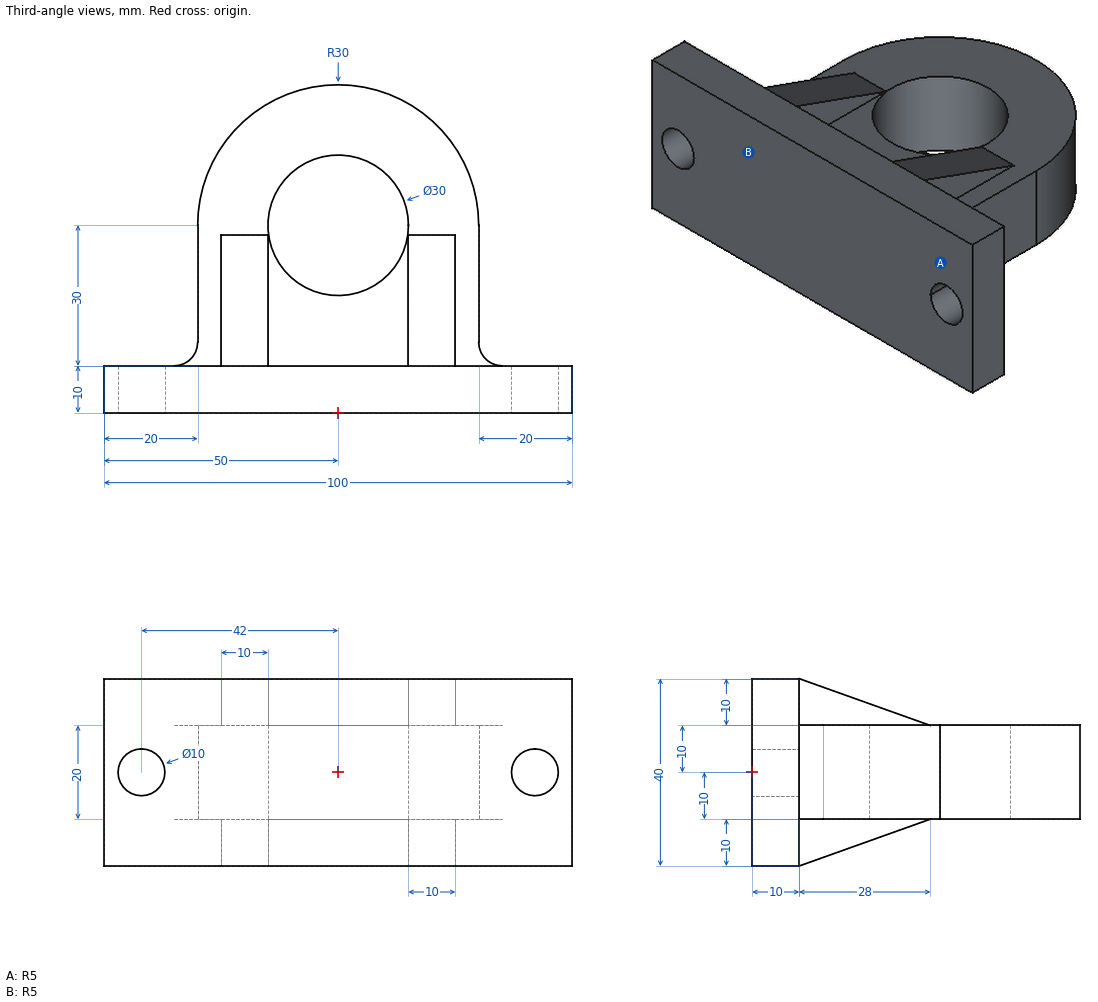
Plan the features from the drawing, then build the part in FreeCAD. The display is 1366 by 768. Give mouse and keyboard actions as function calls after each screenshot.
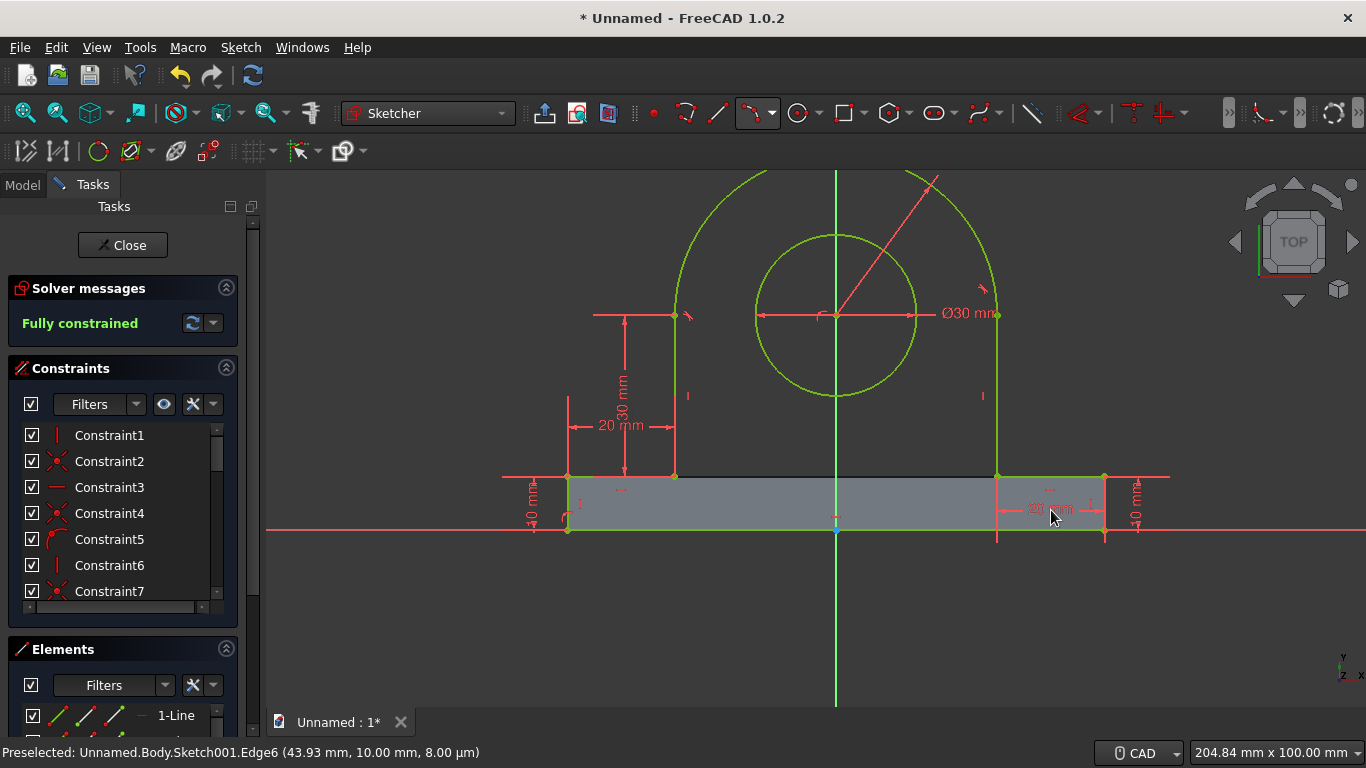
click(123, 245)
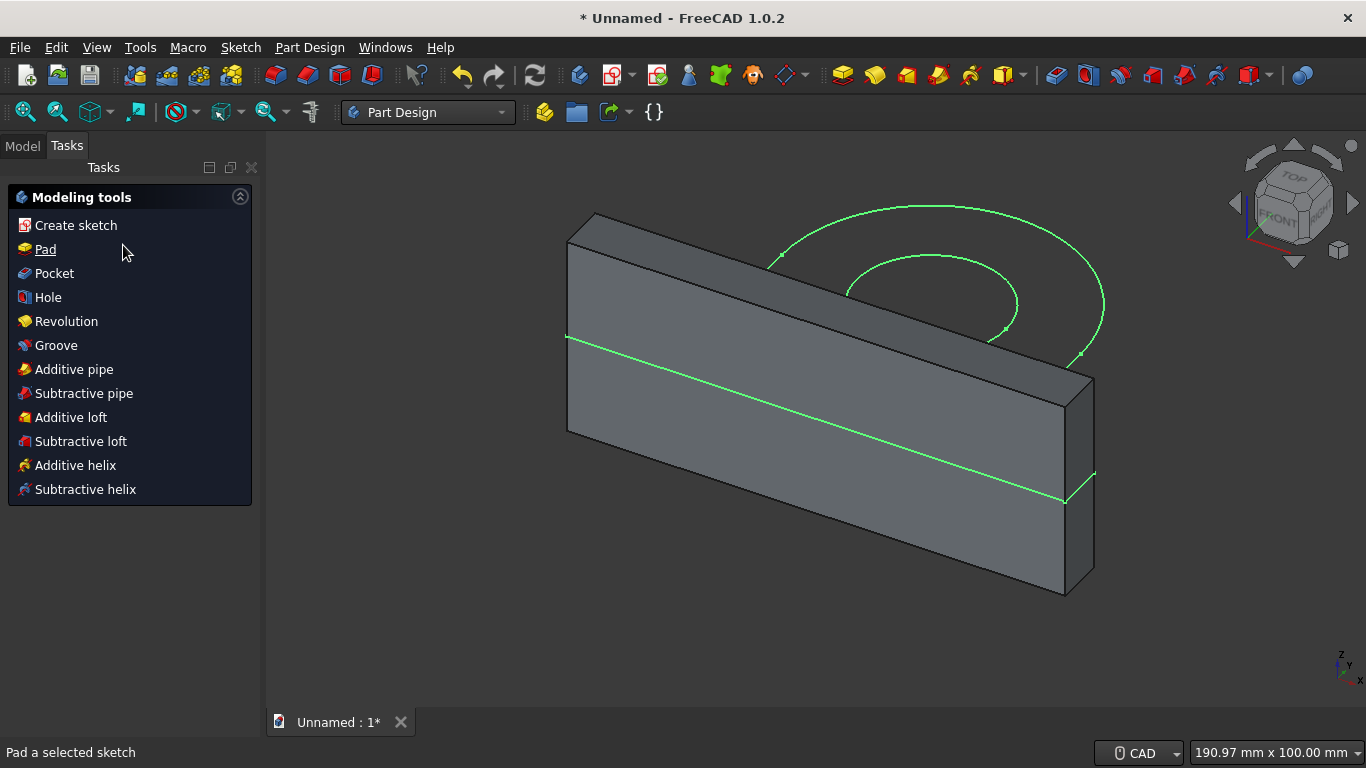
click(844, 76)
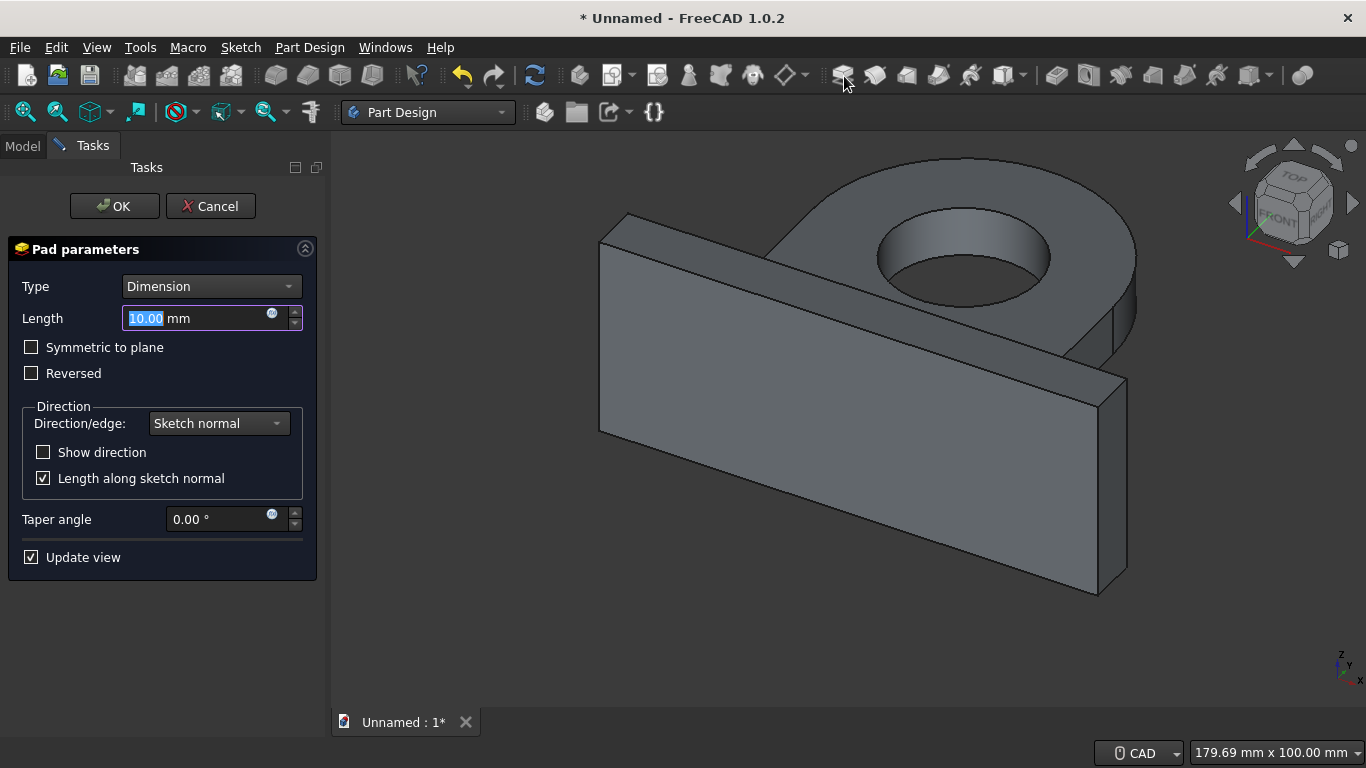
text(20)
key(Tab)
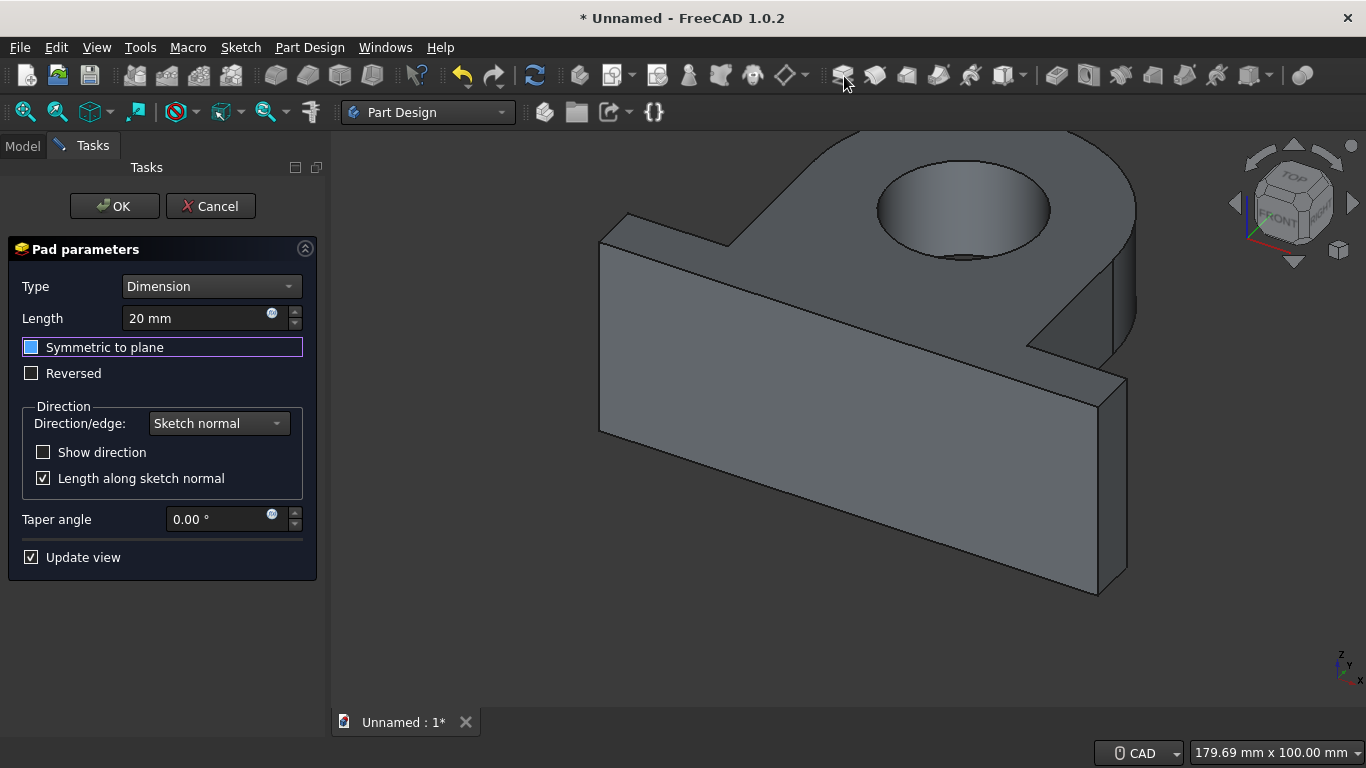
click(30, 347)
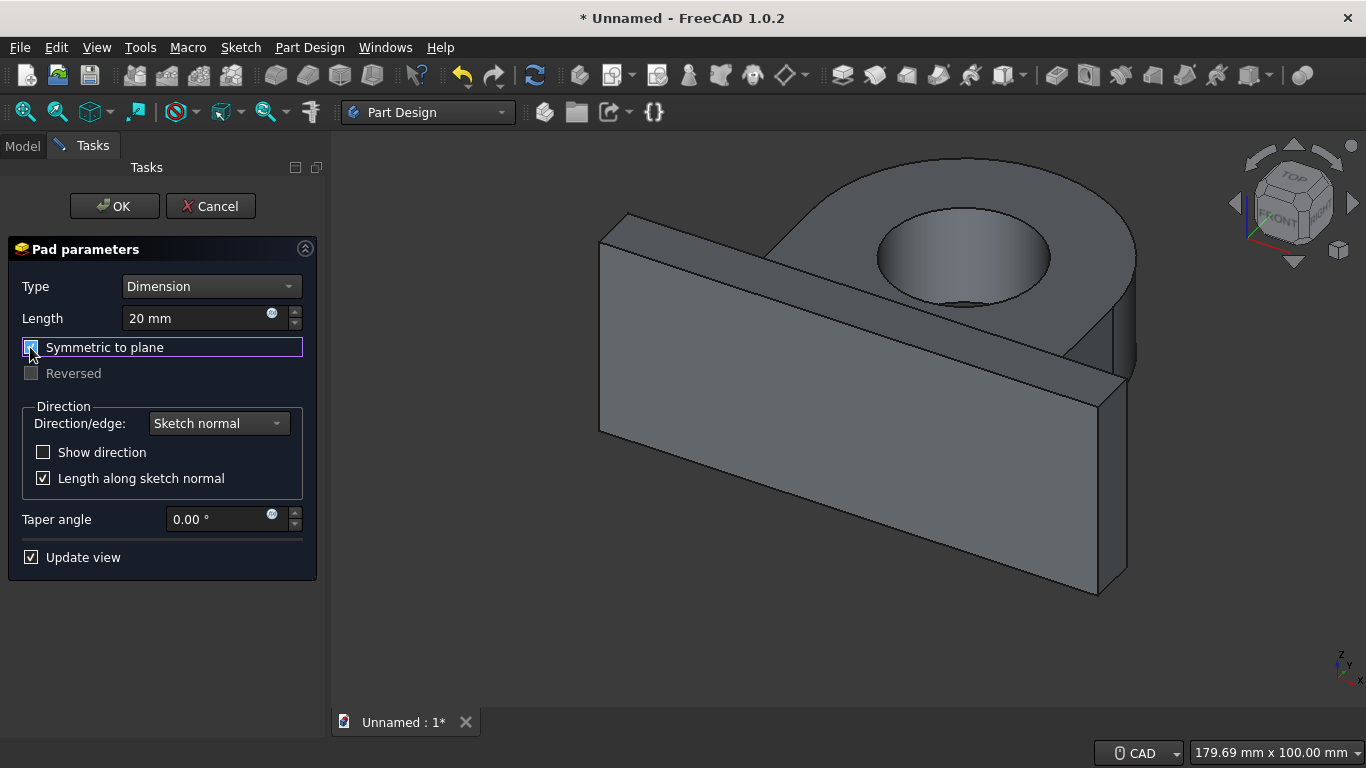
click(115, 206)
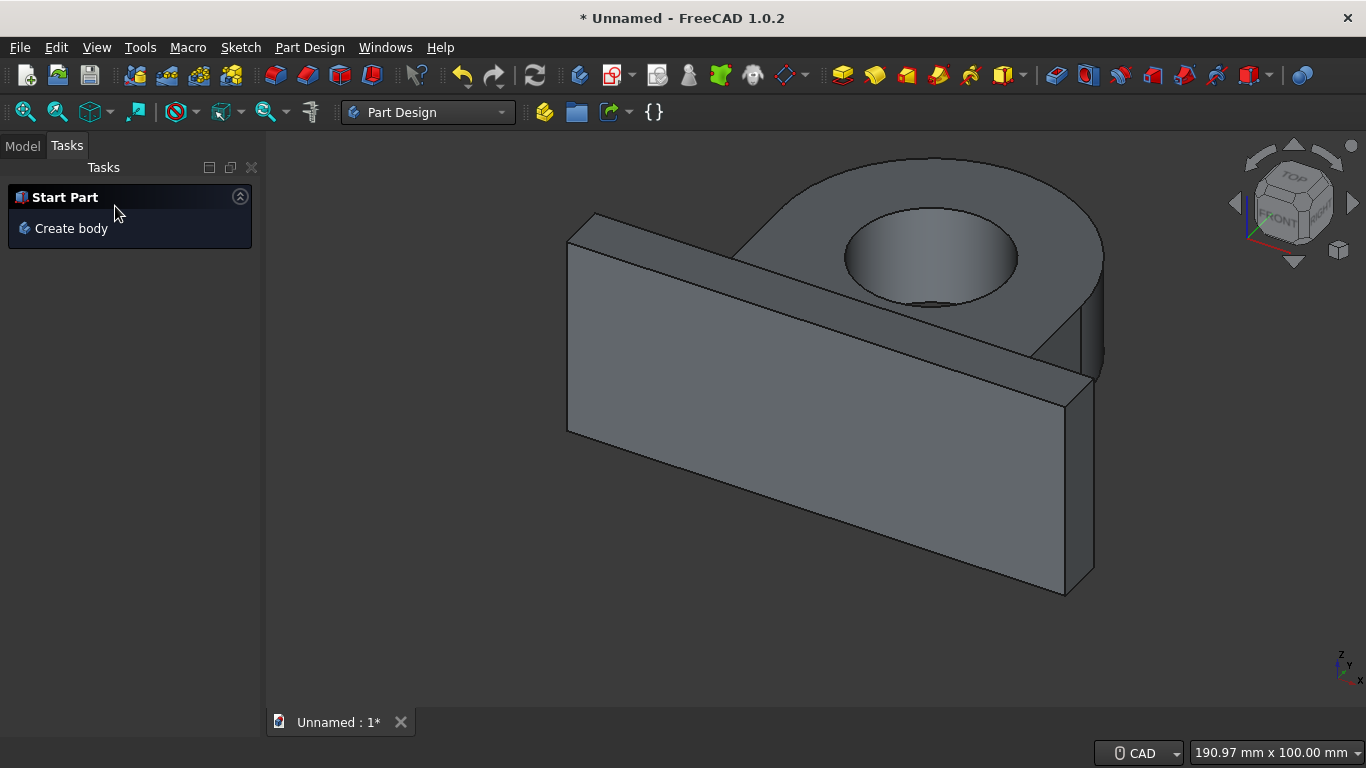
click(26, 112)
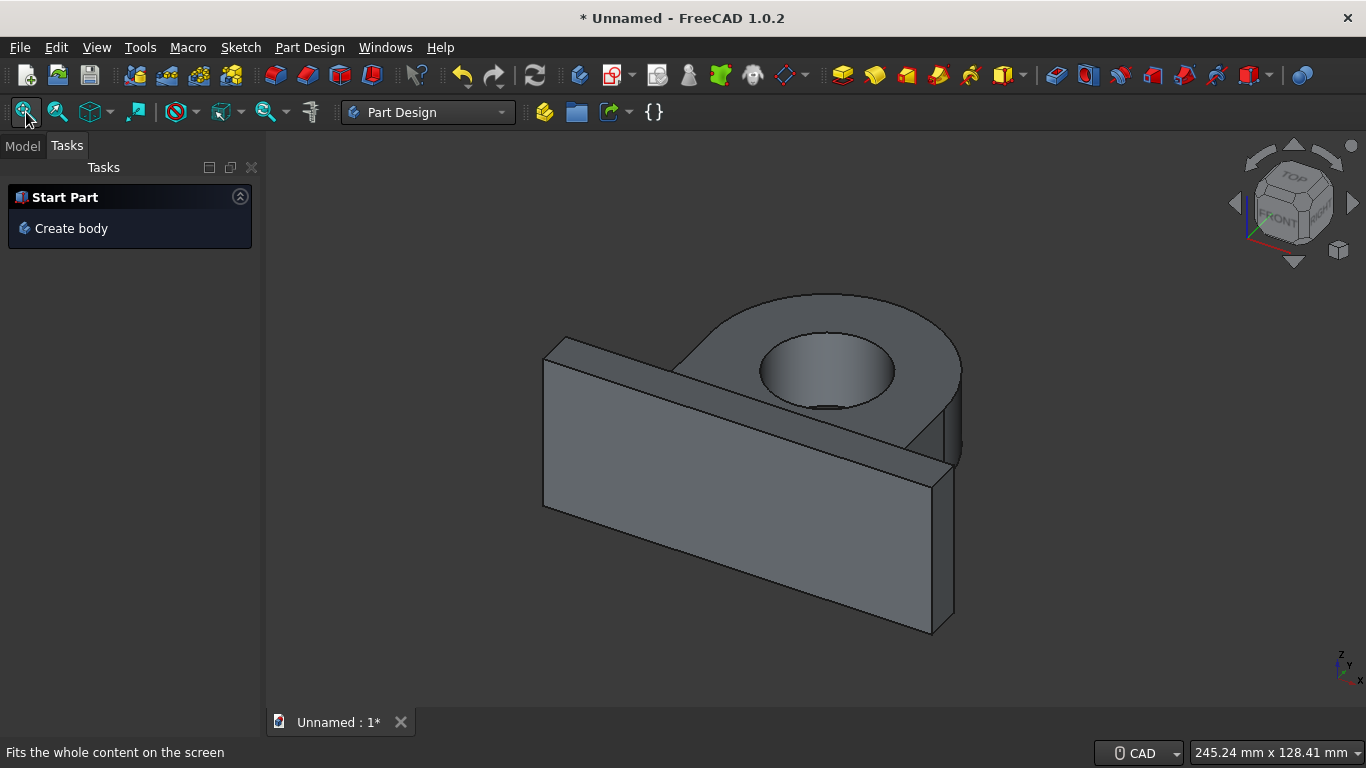
key(0)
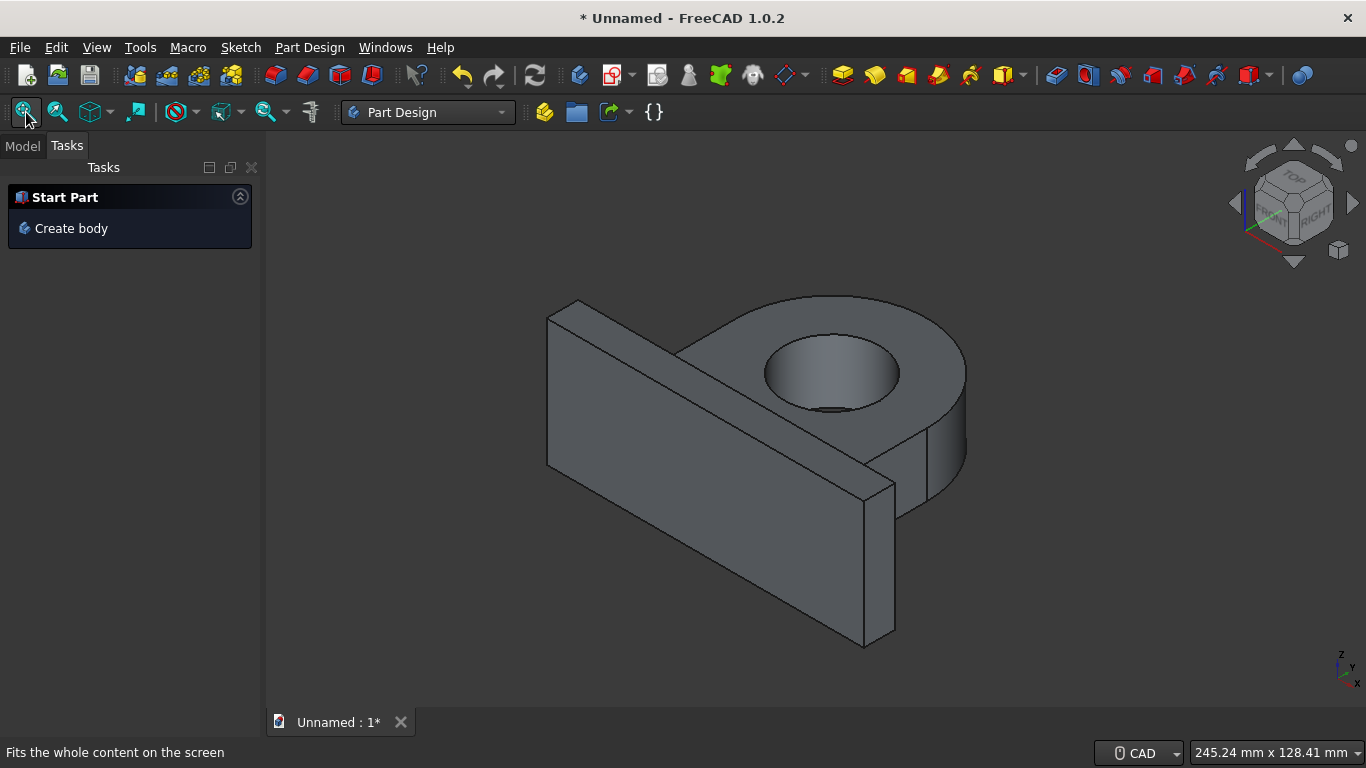
key(2)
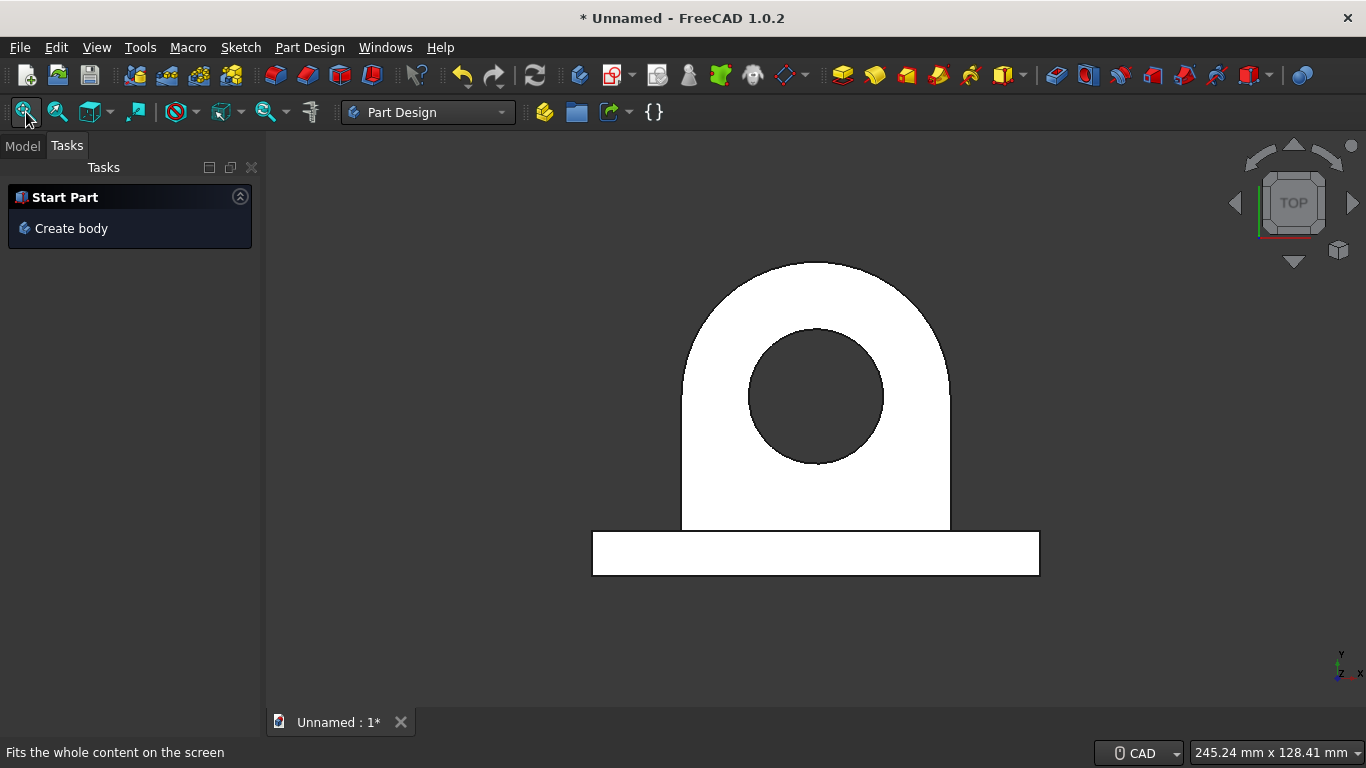
key(1)